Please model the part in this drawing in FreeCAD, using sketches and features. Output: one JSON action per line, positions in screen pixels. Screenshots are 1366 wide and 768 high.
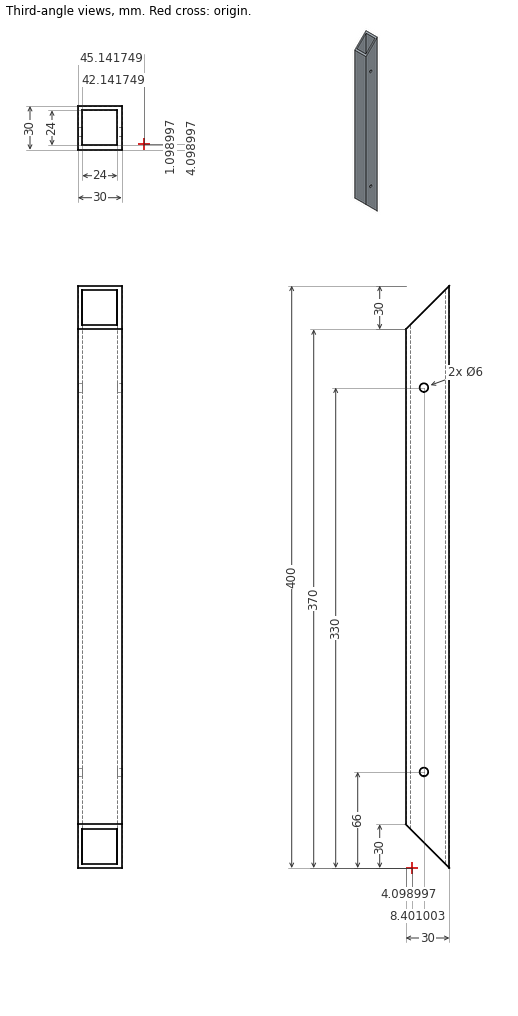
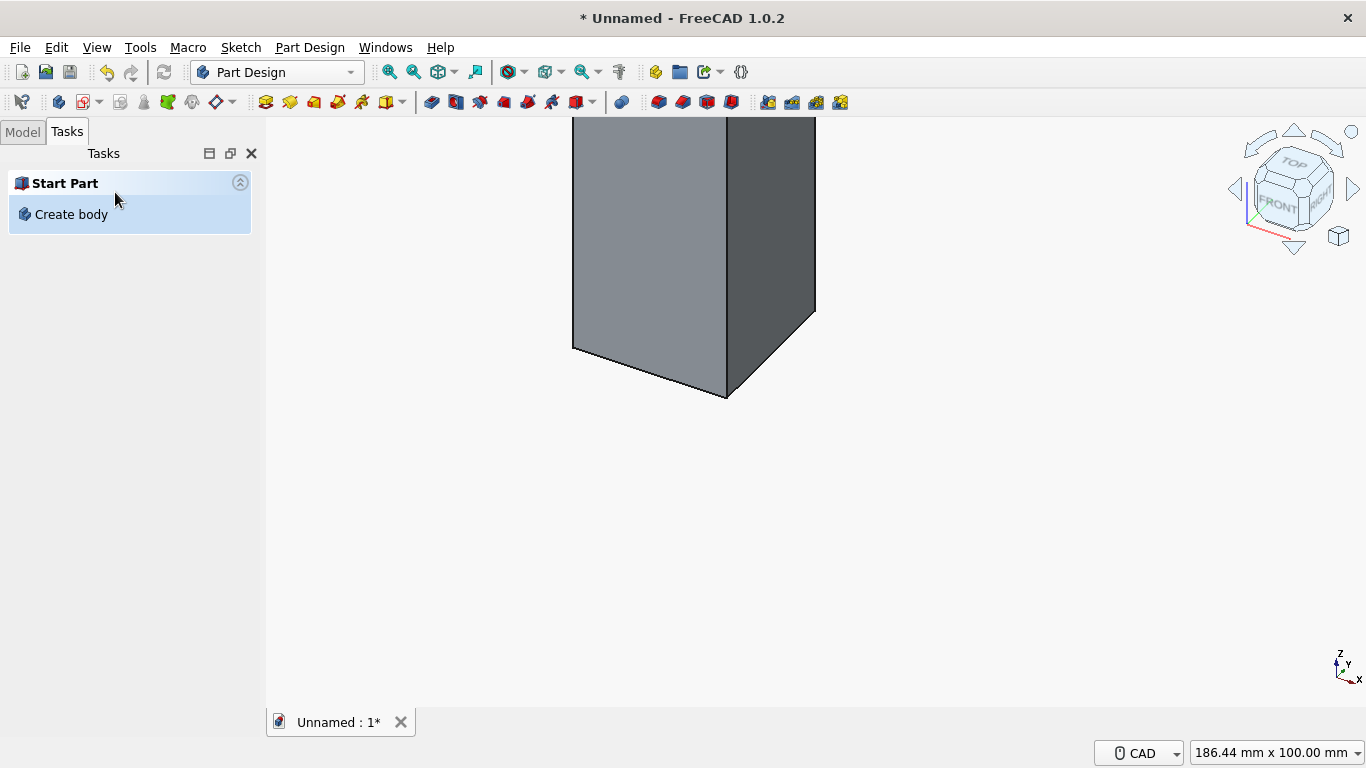
{"action": "left_click", "coordinate": [390, 72]}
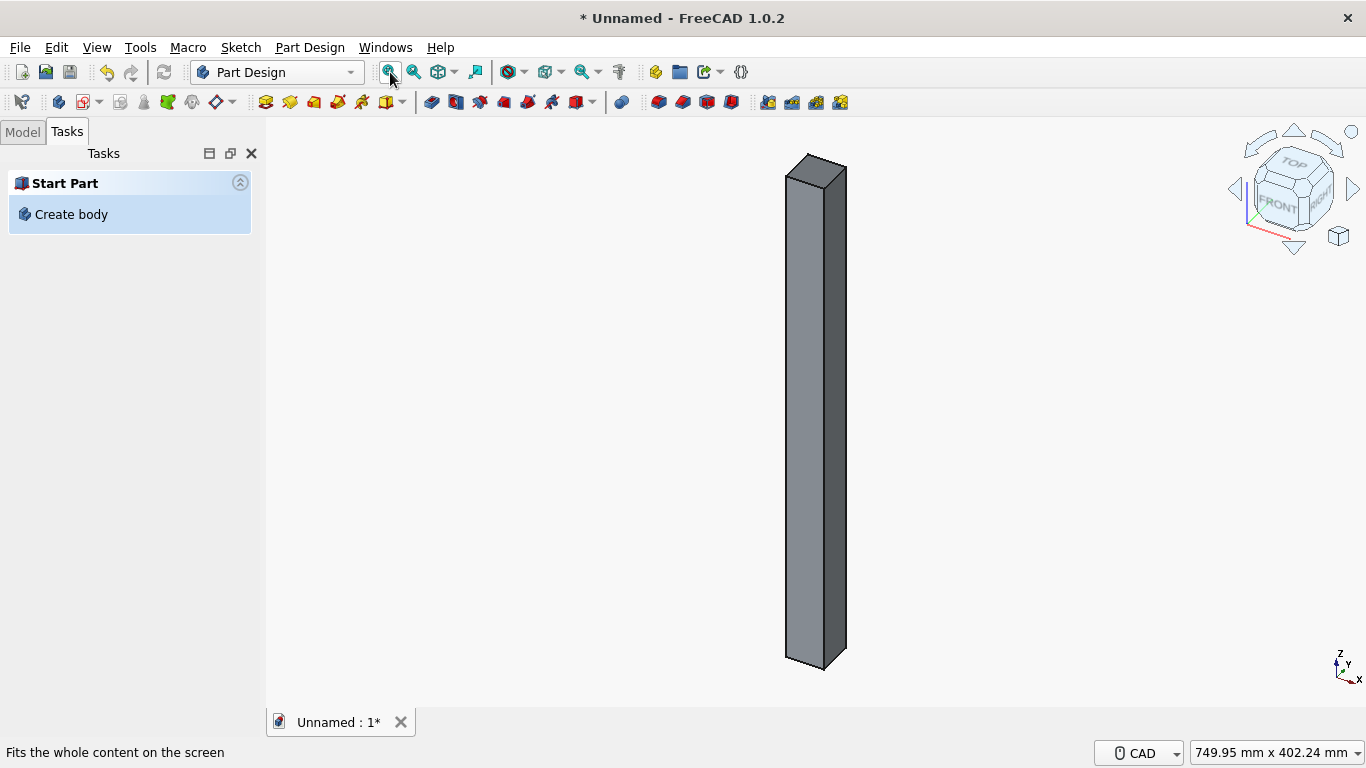
{"action": "left_click", "coordinate": [816, 171]}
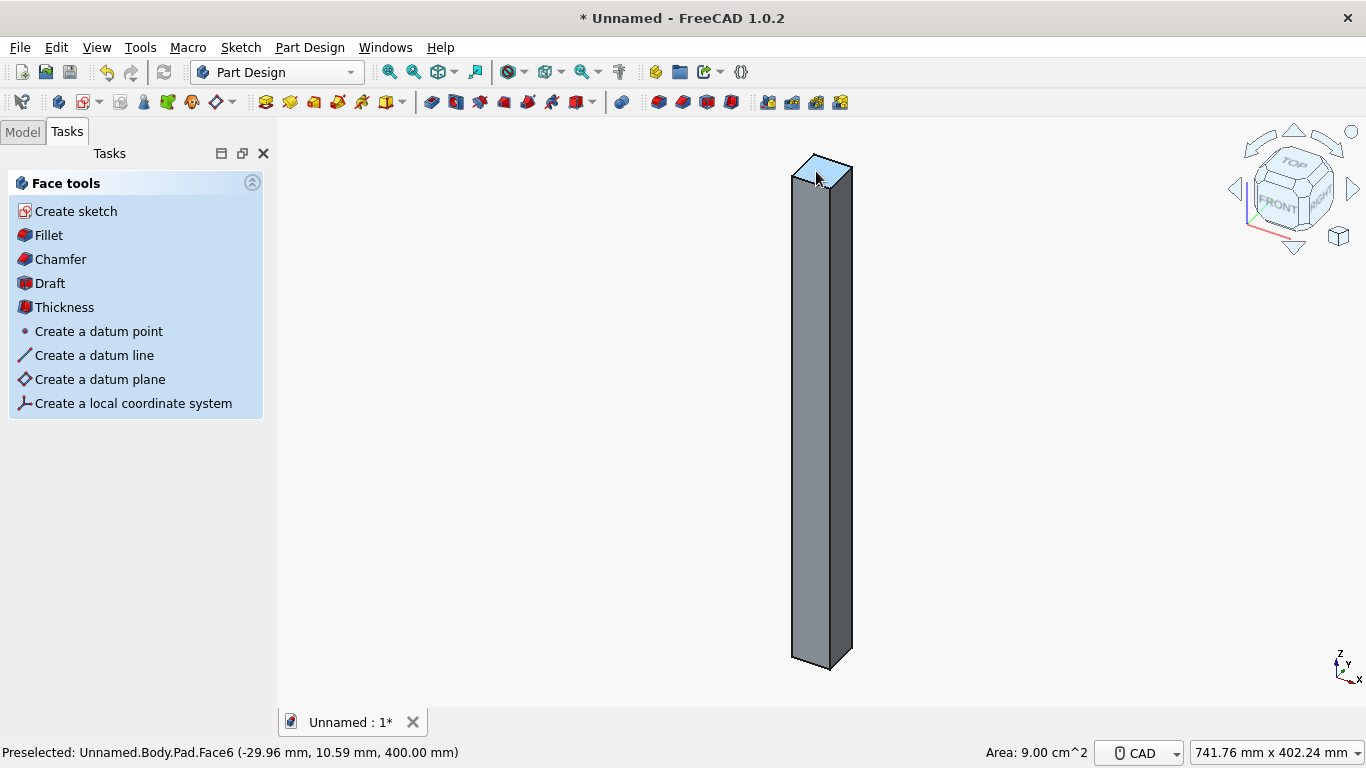
{"action": "left_click", "coordinate": [84, 102]}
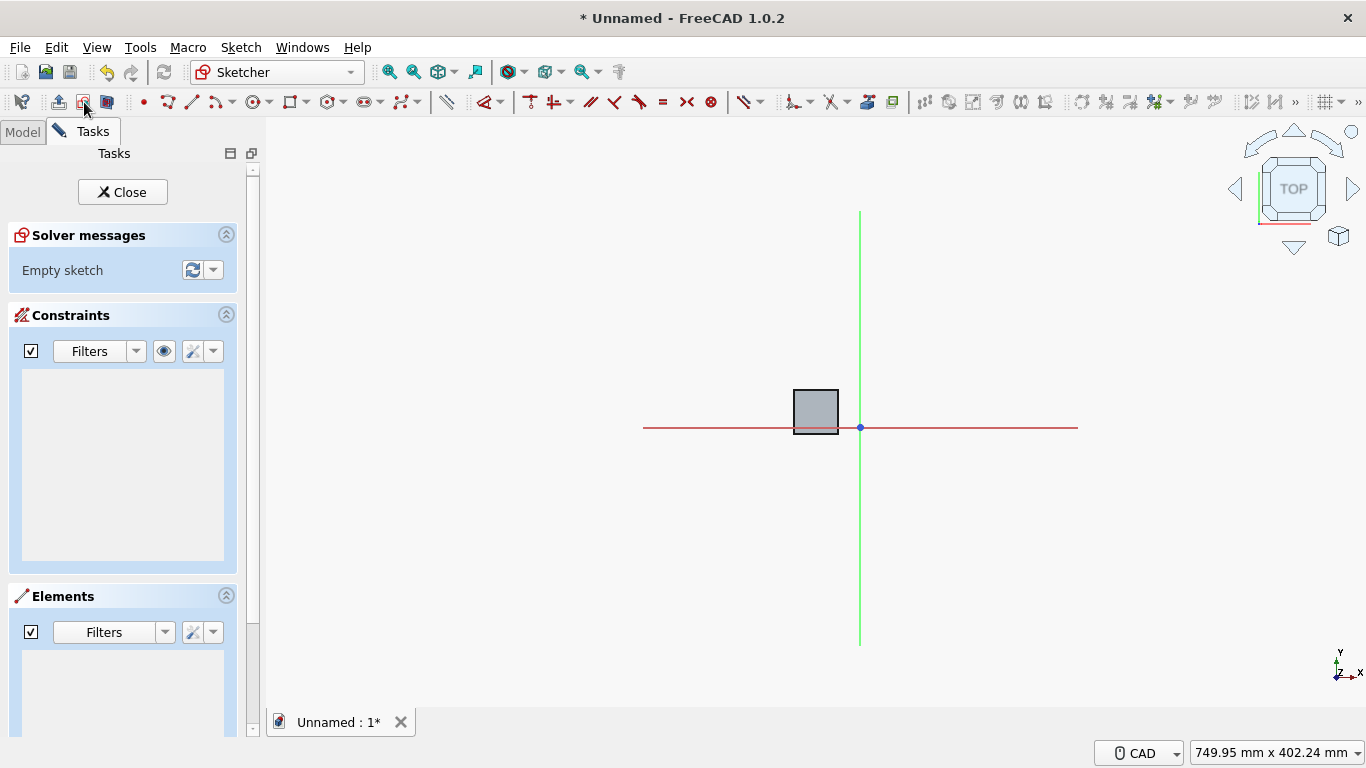
{"action": "scroll", "coordinate": [837, 412], "scroll_direction": "up", "scroll_amount": 12}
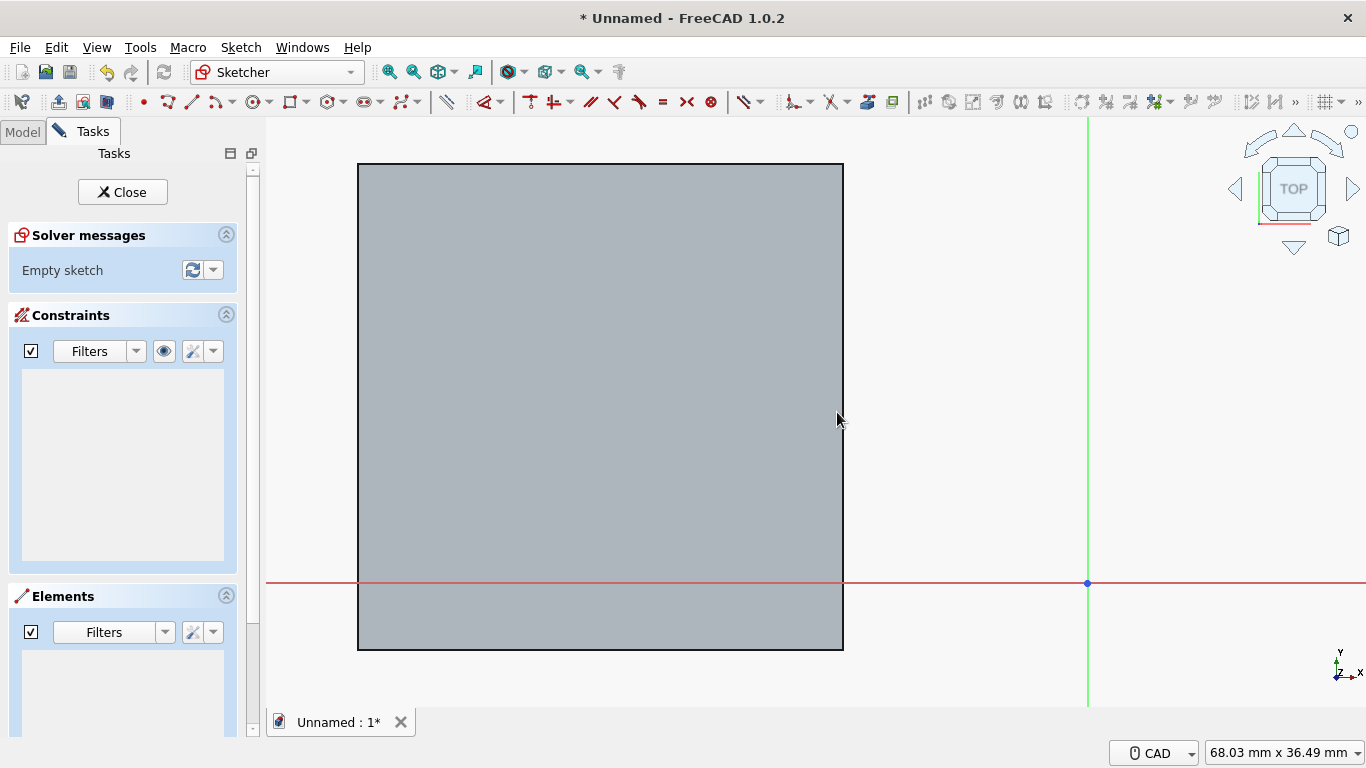
{"action": "left_click", "coordinate": [290, 102]}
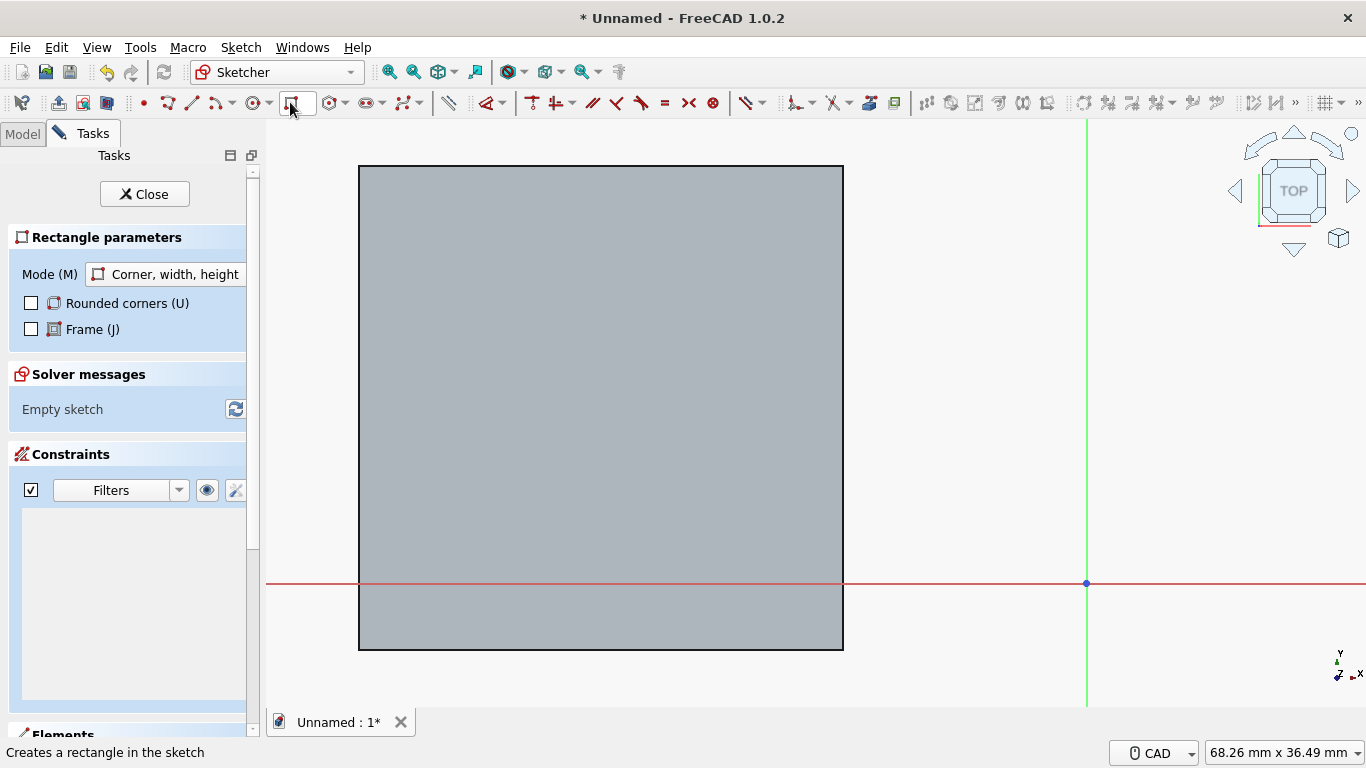
{"action": "left_click", "coordinate": [408, 215]}
{"action": "left_click", "coordinate": [794, 601]}
{"action": "key", "text": "Escape"}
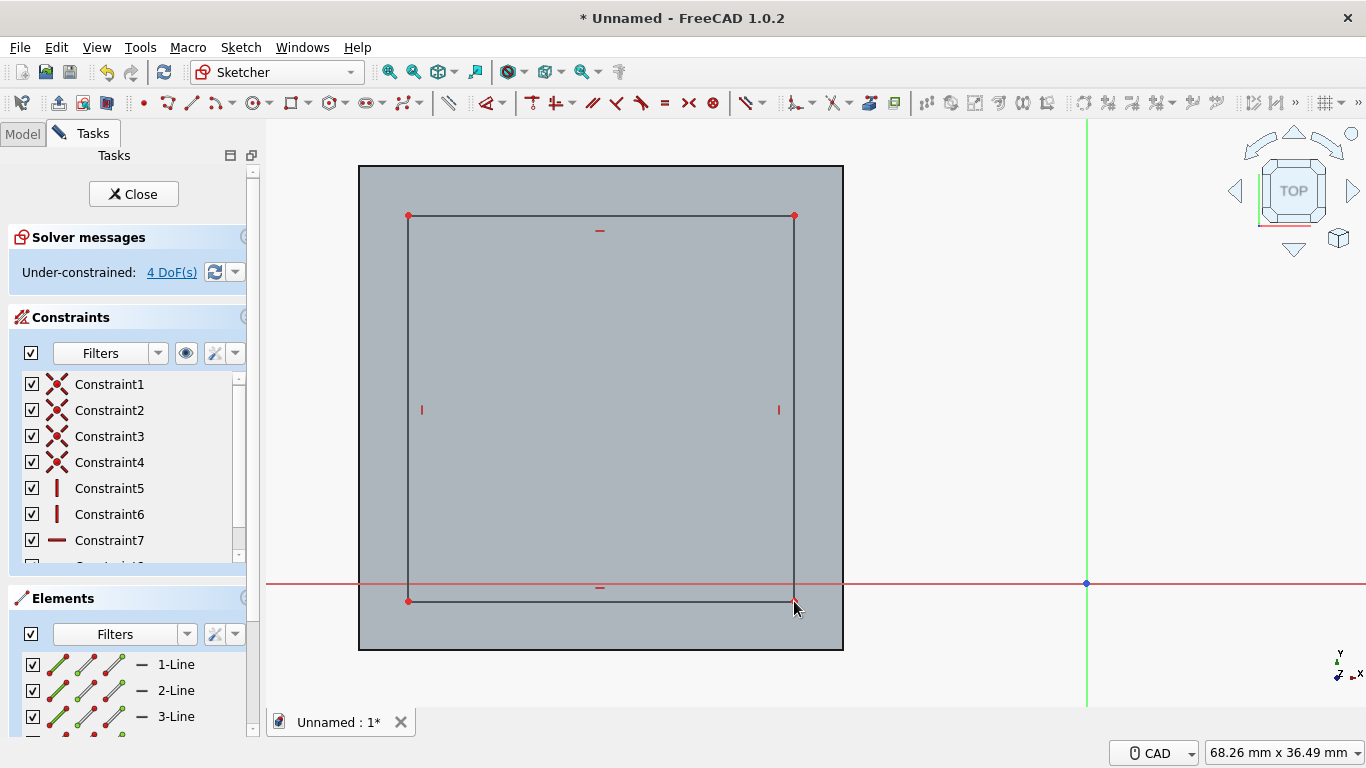
{"action": "left_click", "coordinate": [486, 104]}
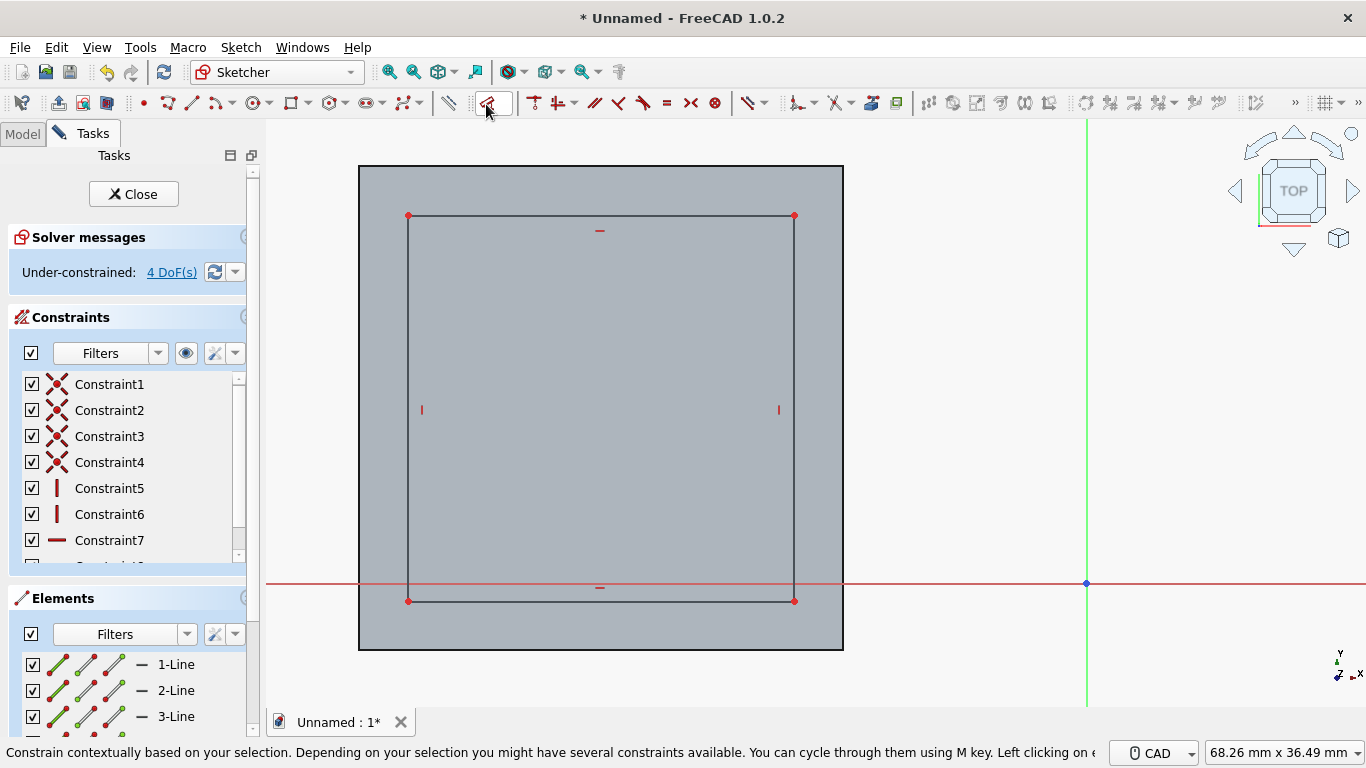
{"action": "left_click", "coordinate": [408, 332]}
{"action": "left_click", "coordinate": [374, 409]}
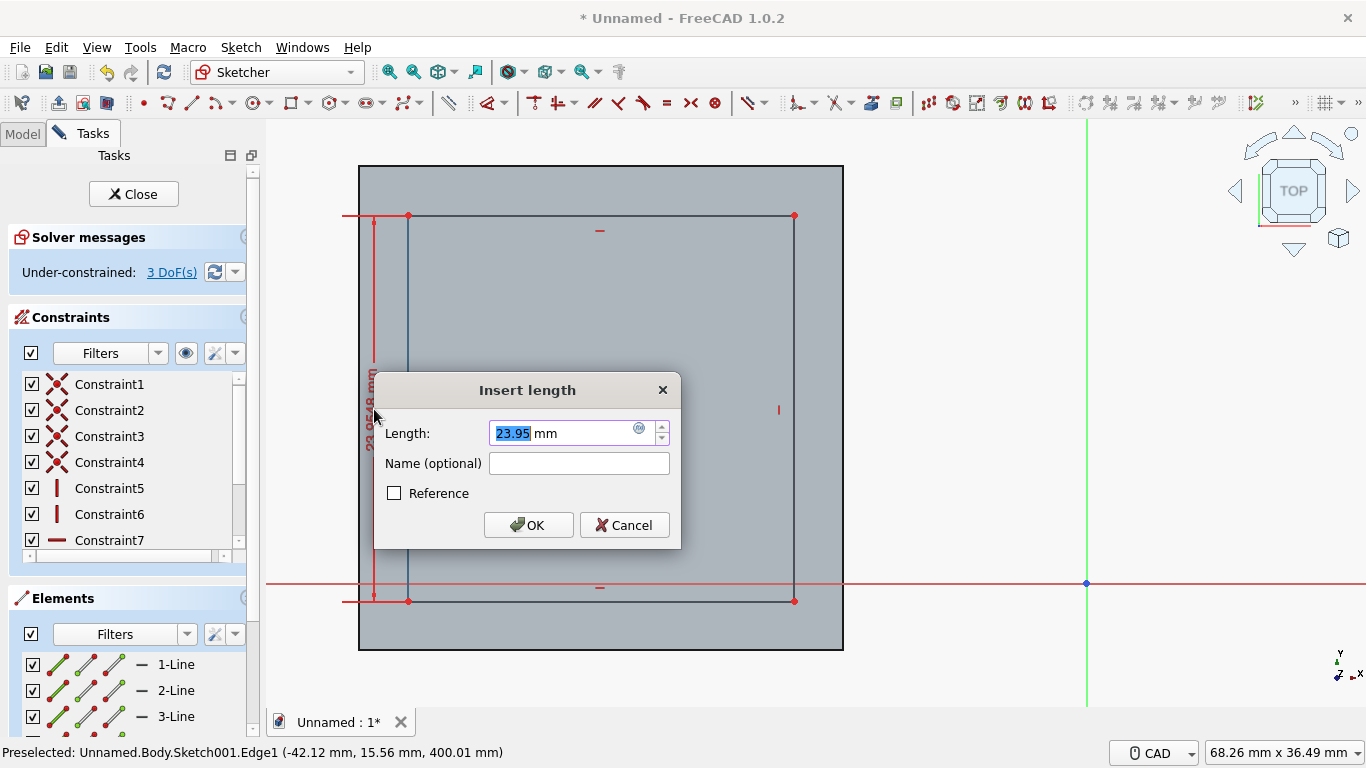
{"action": "type", "text": "24"}
{"action": "key", "text": "Return"}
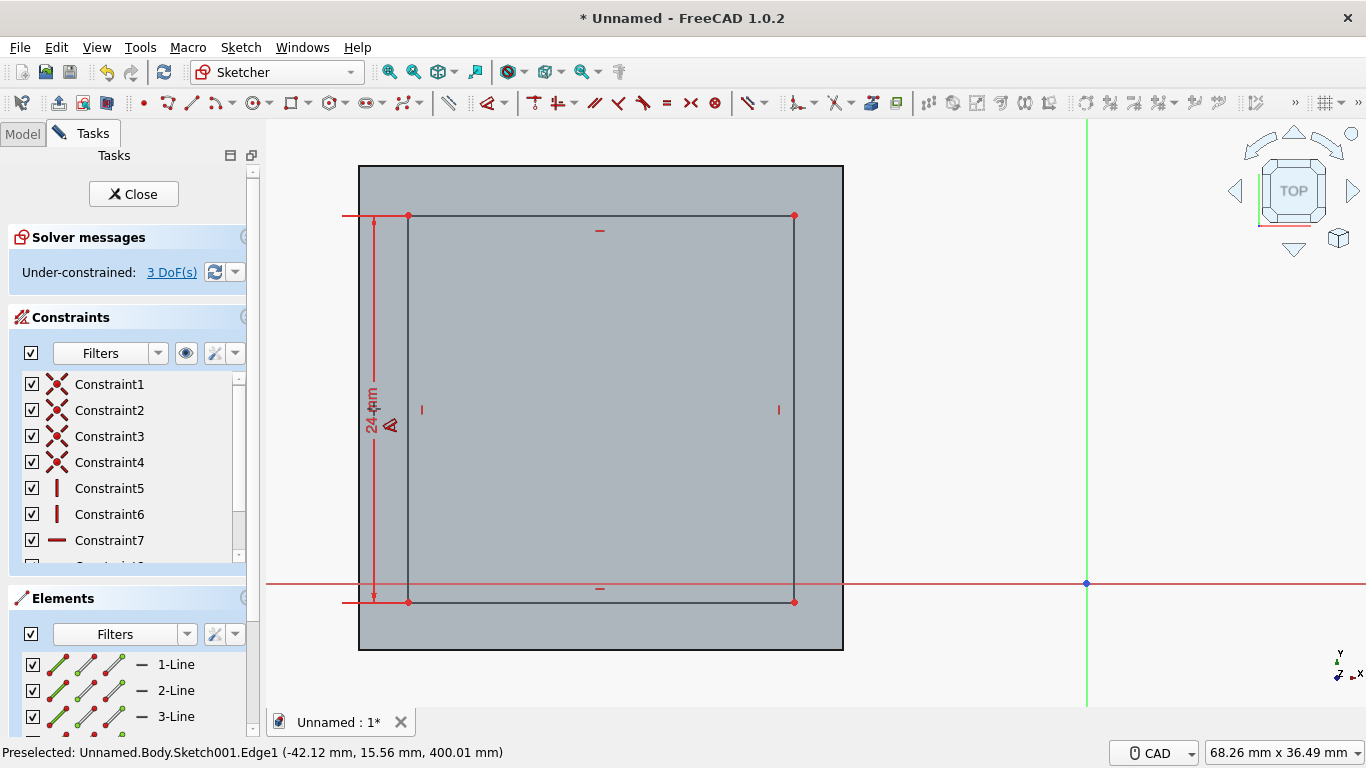
{"action": "left_click", "coordinate": [524, 603]}
{"action": "left_click", "coordinate": [601, 637]}